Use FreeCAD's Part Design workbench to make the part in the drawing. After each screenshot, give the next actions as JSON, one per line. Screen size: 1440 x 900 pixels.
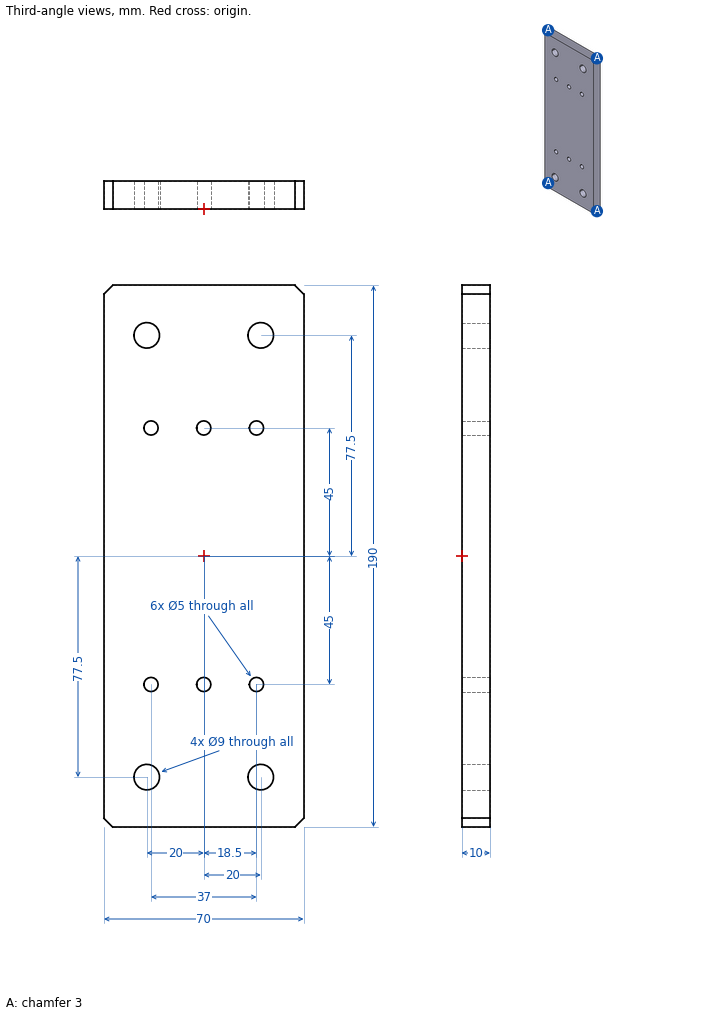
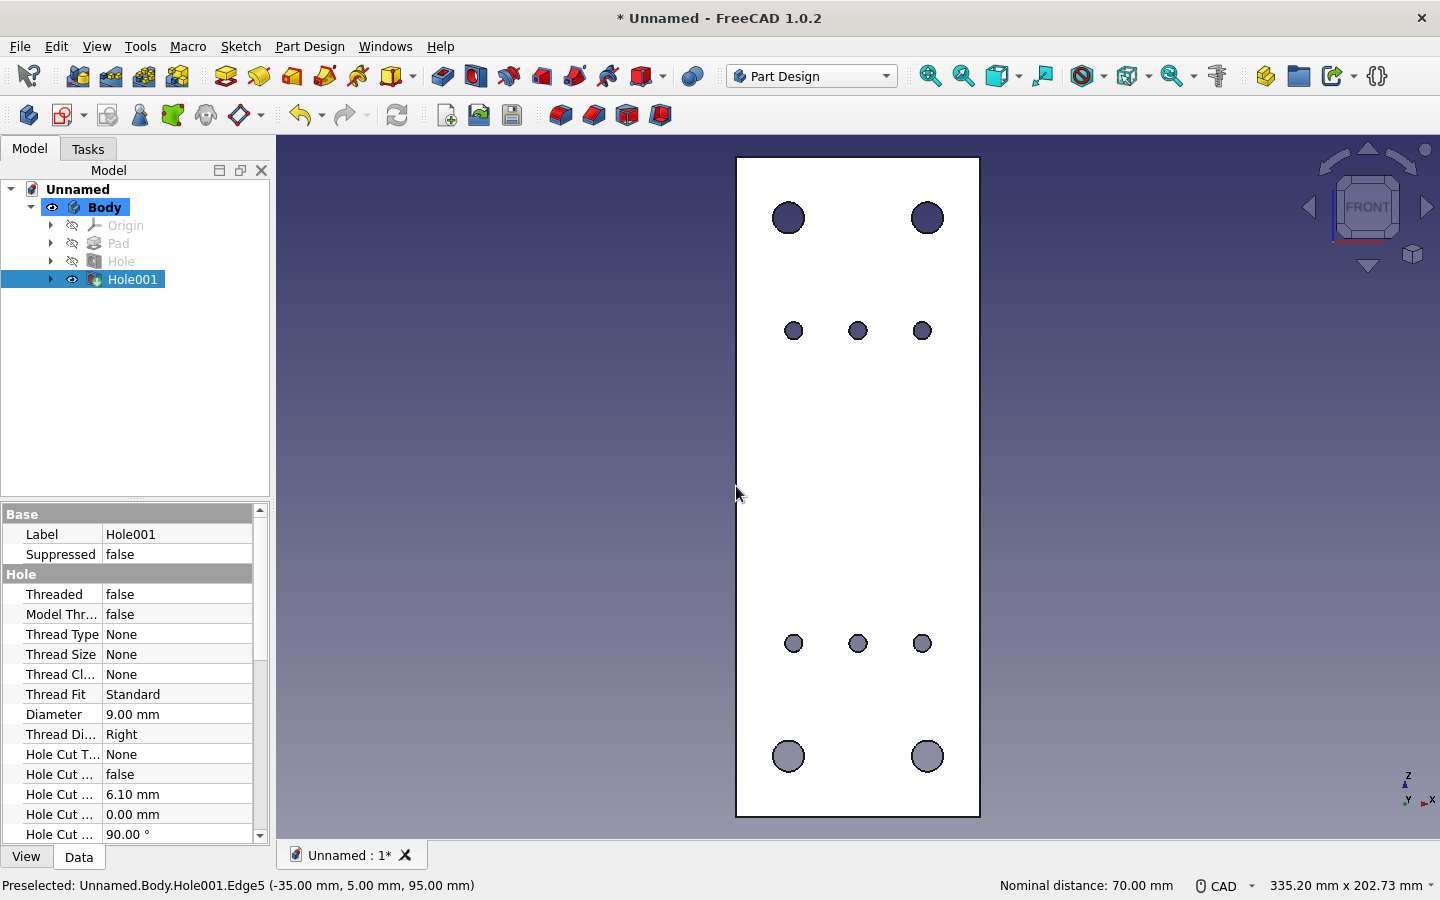
{"action": "key", "text": "3"}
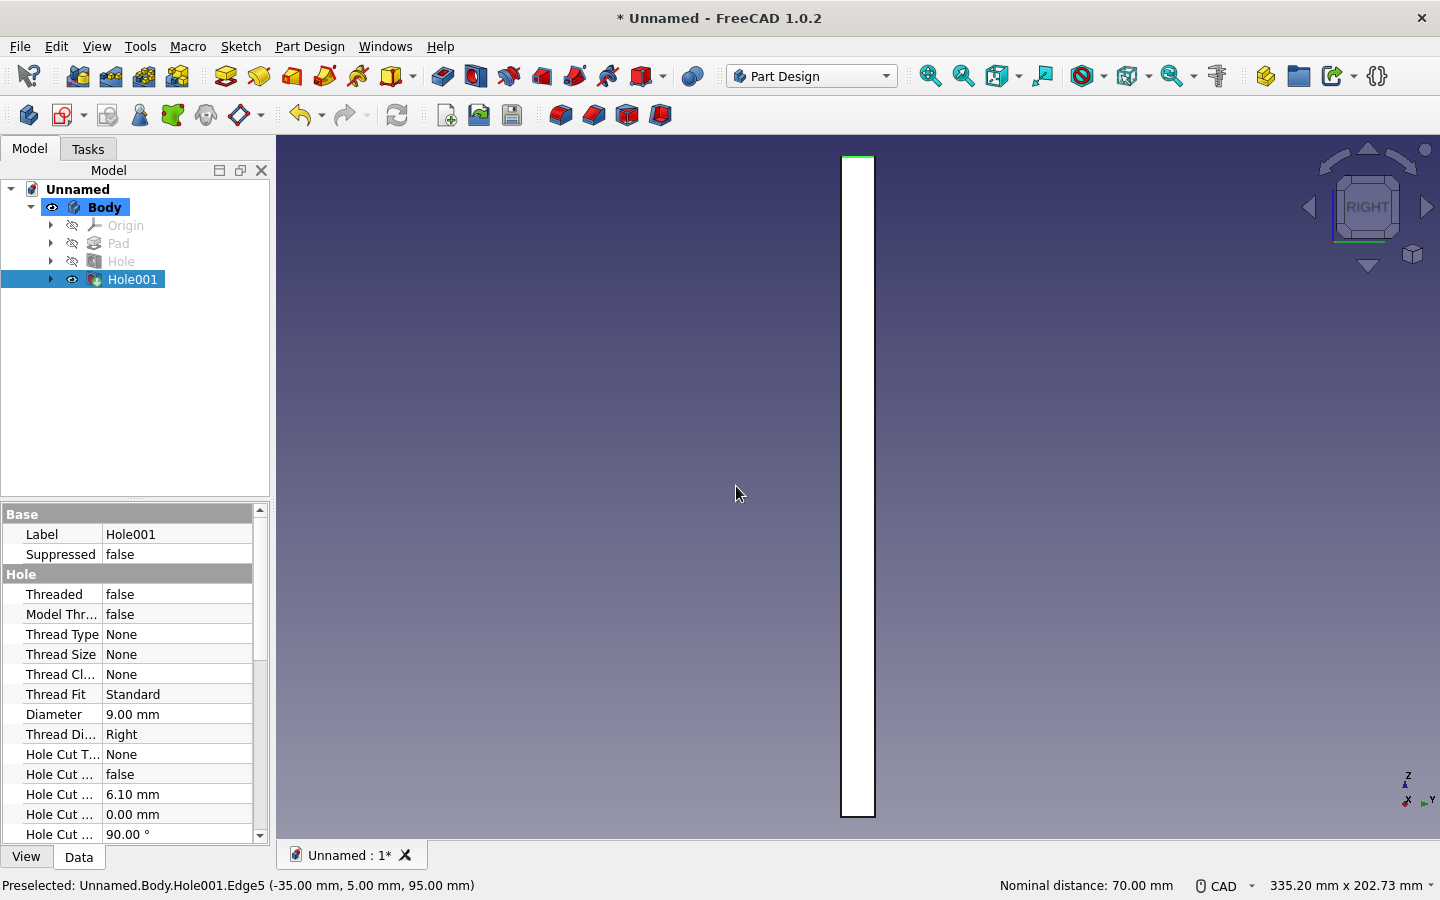
{"action": "key", "text": "5"}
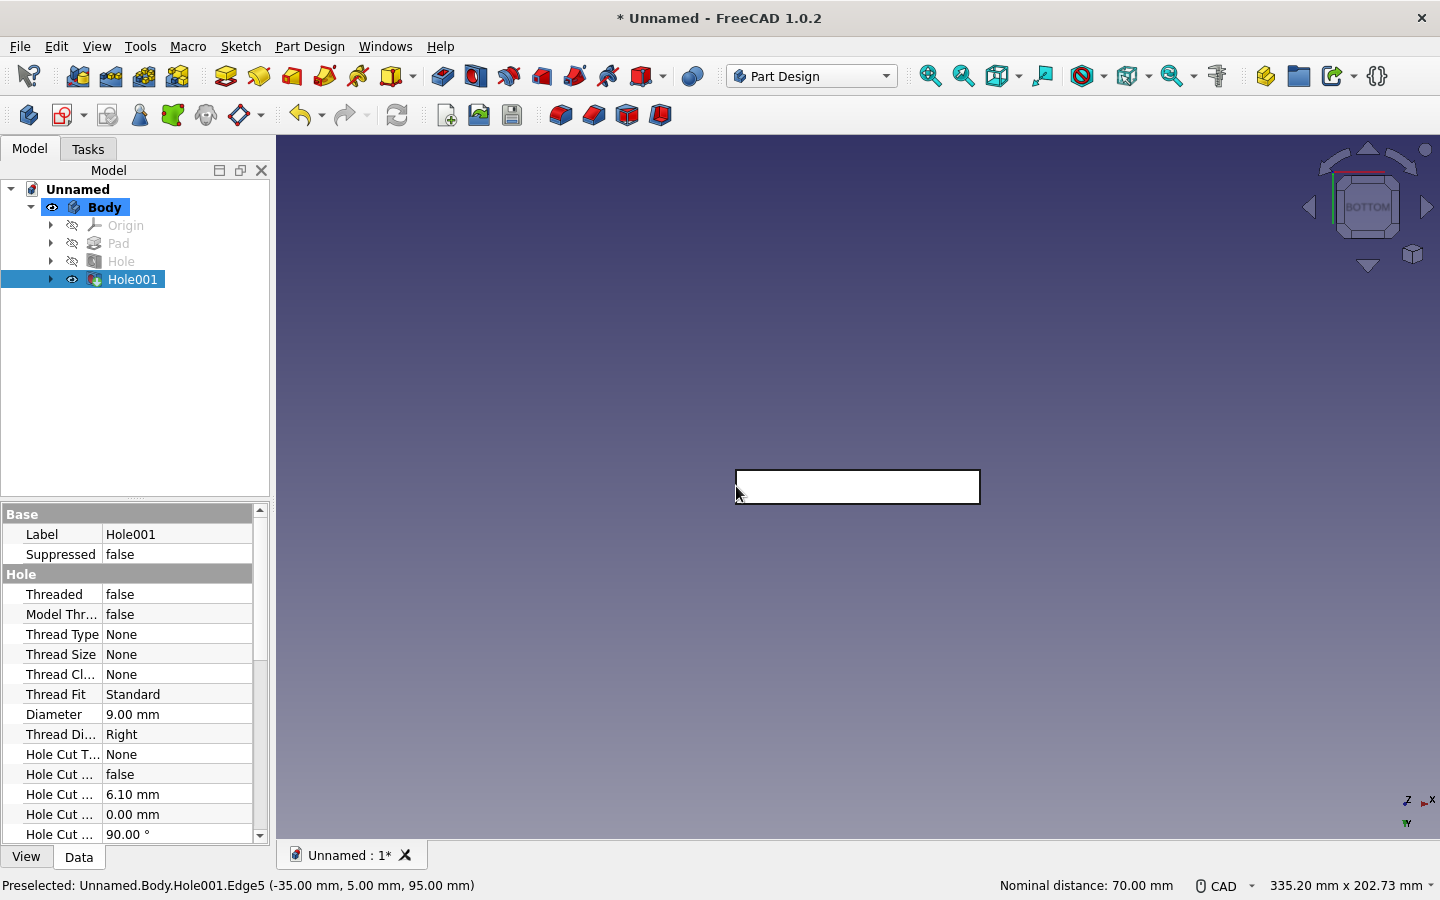
{"action": "left_click", "coordinate": [931, 76]}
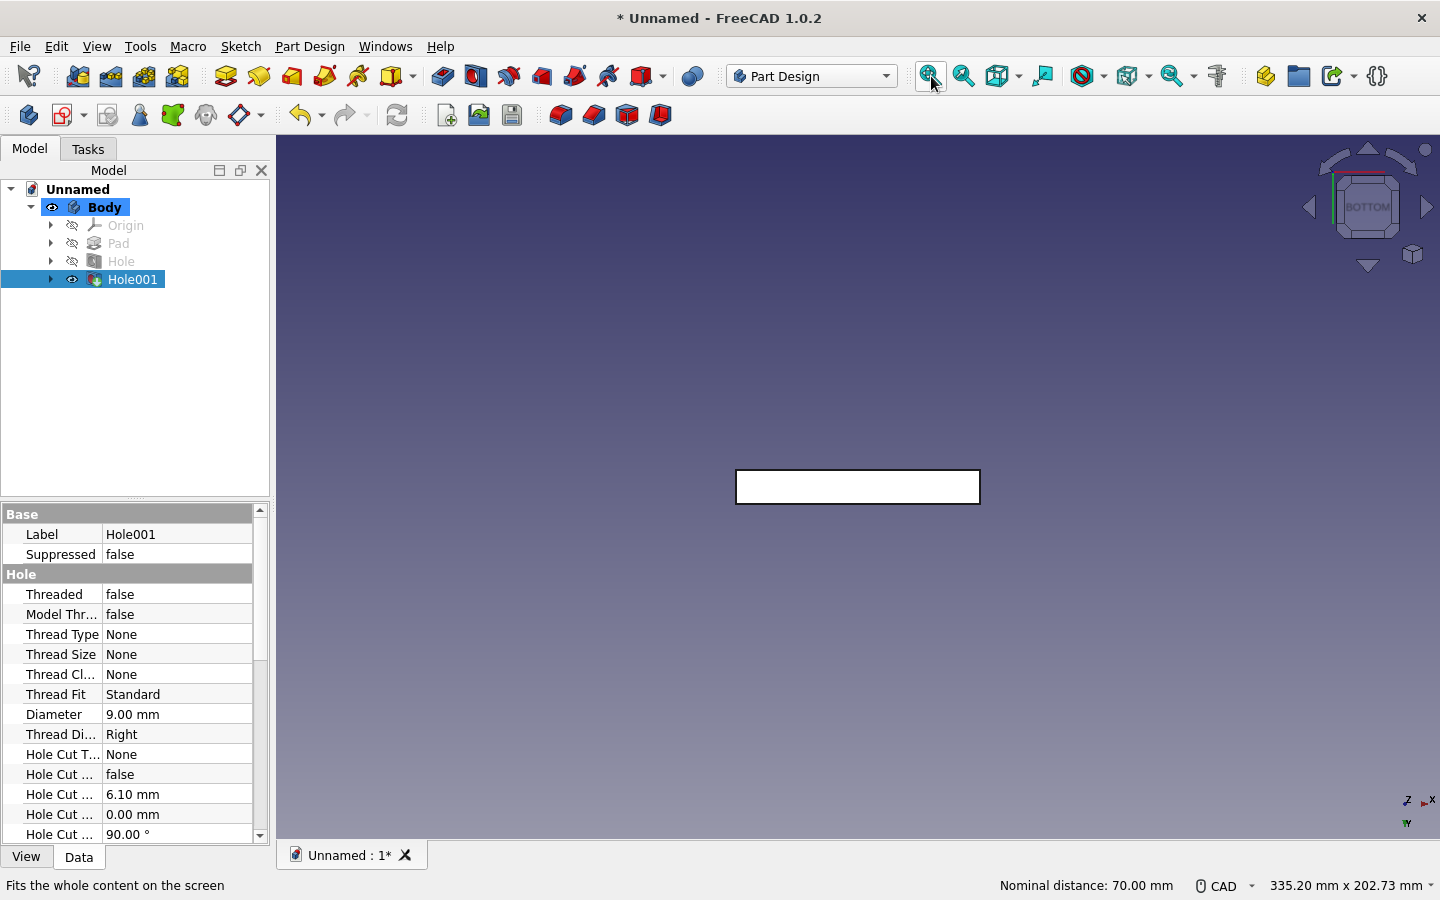
{"action": "left_click", "coordinate": [736, 486], "text": "ctrl"}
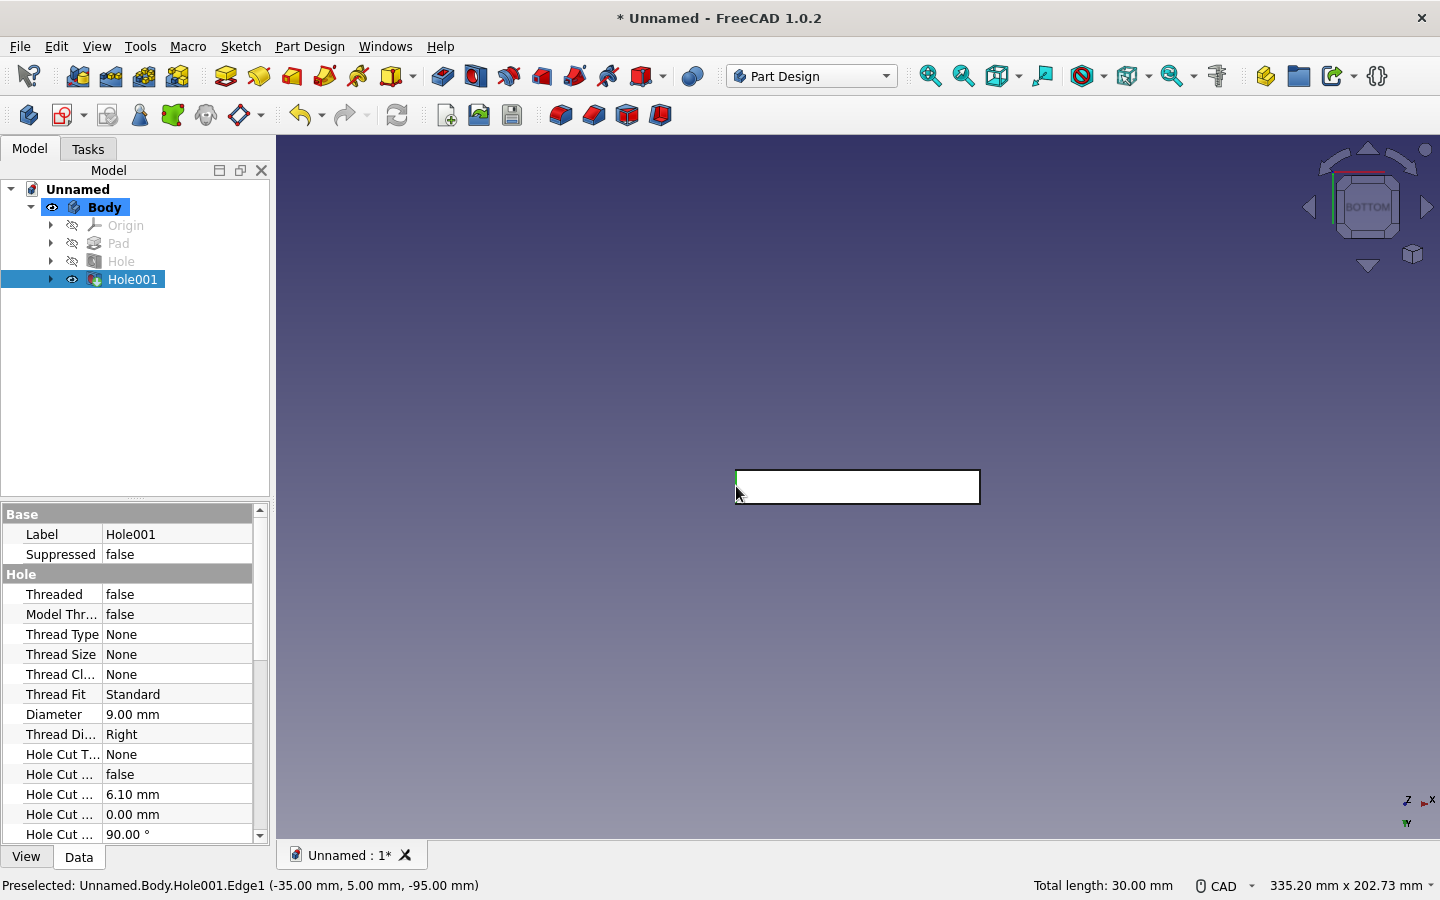
{"action": "left_click", "coordinate": [980, 486], "text": "ctrl"}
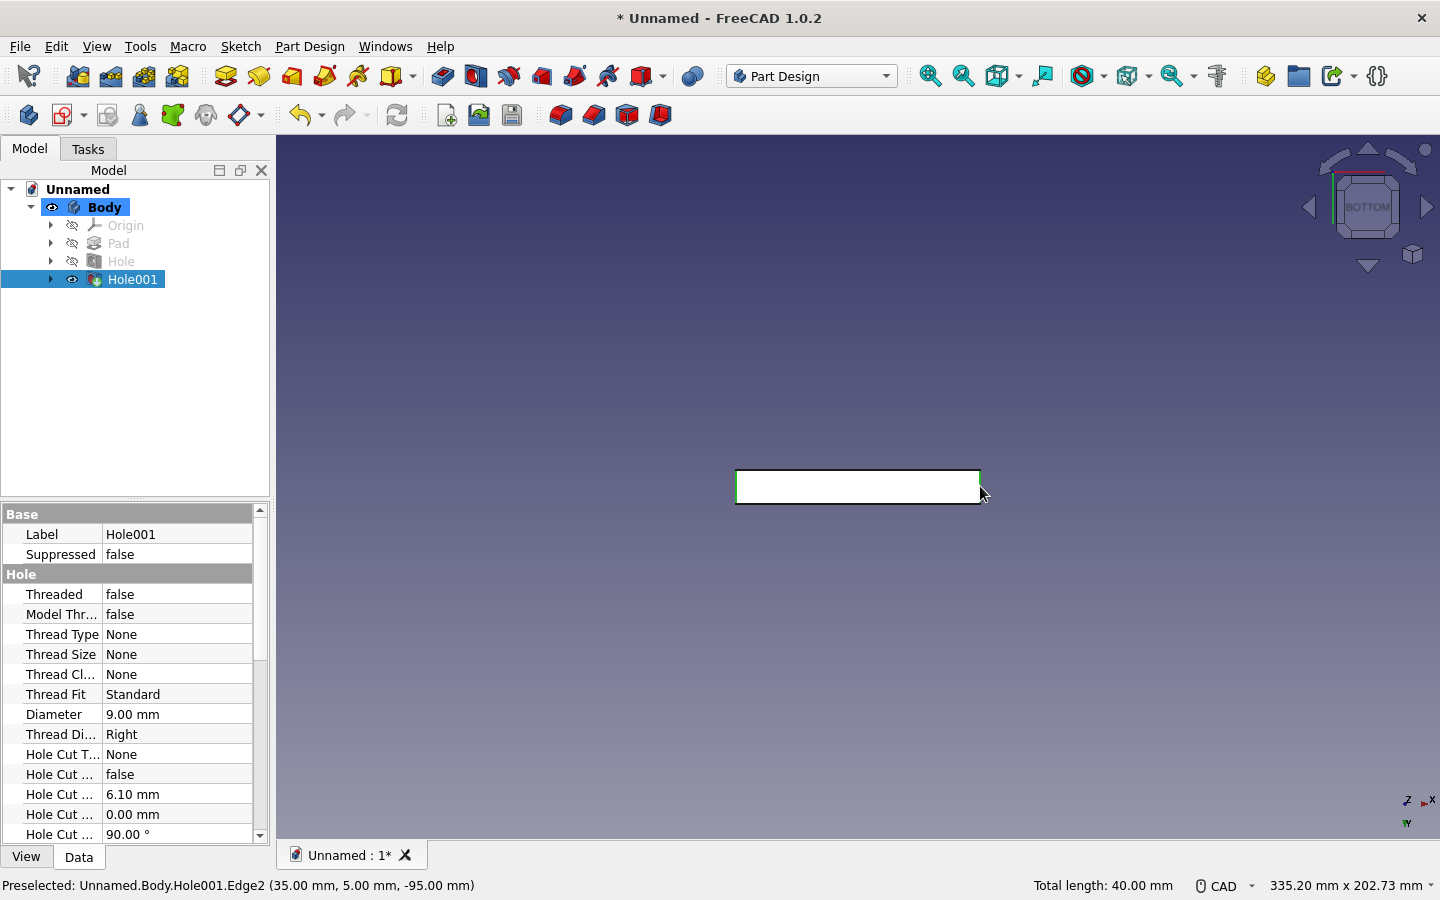
{"action": "left_click", "coordinate": [594, 116]}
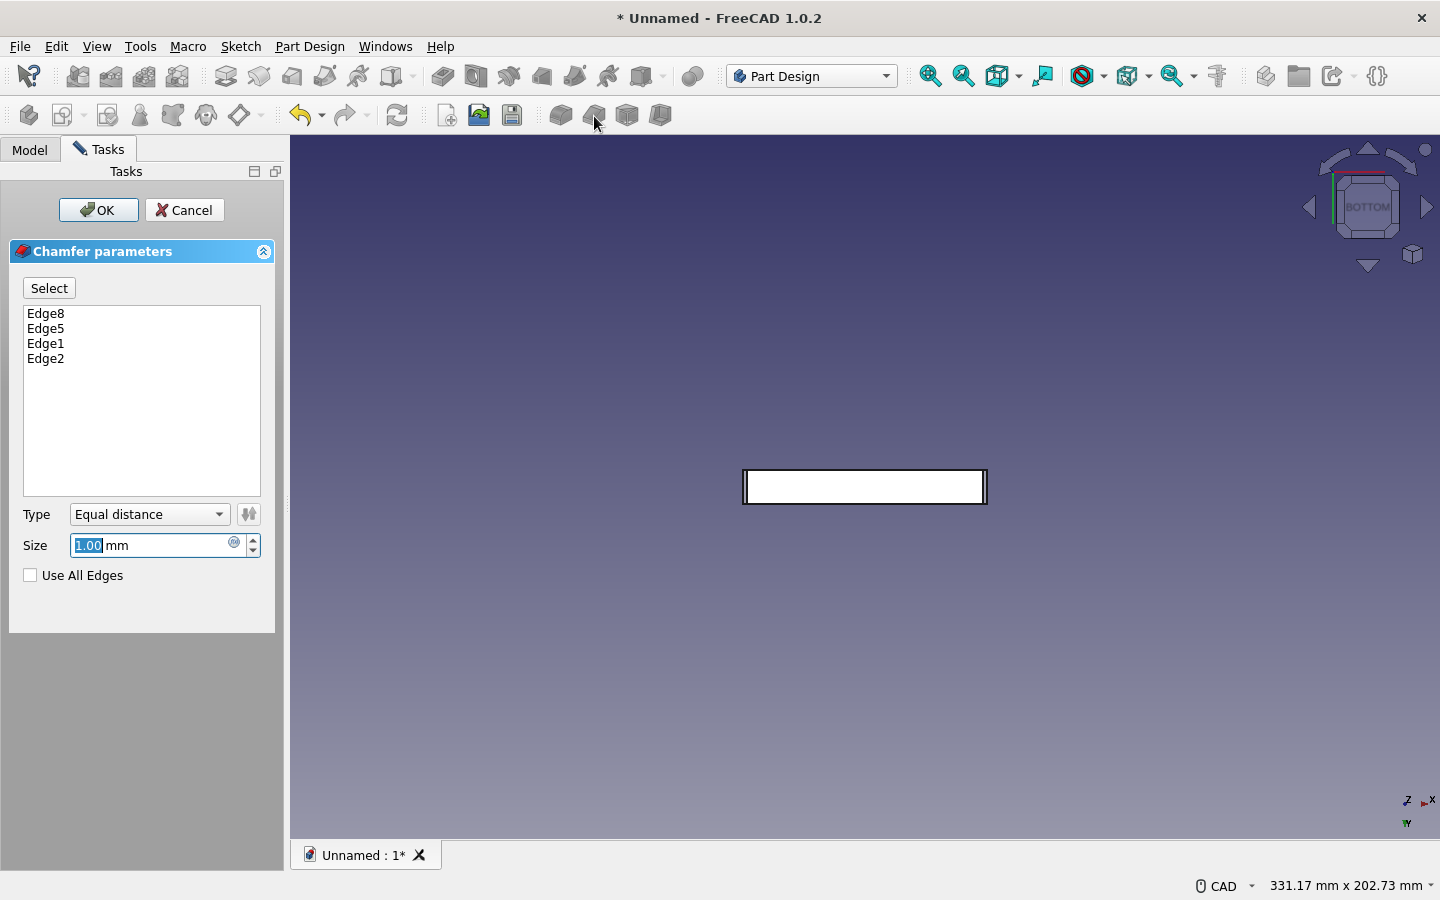
{"action": "type", "text": "3"}
{"action": "key", "text": "Tab"}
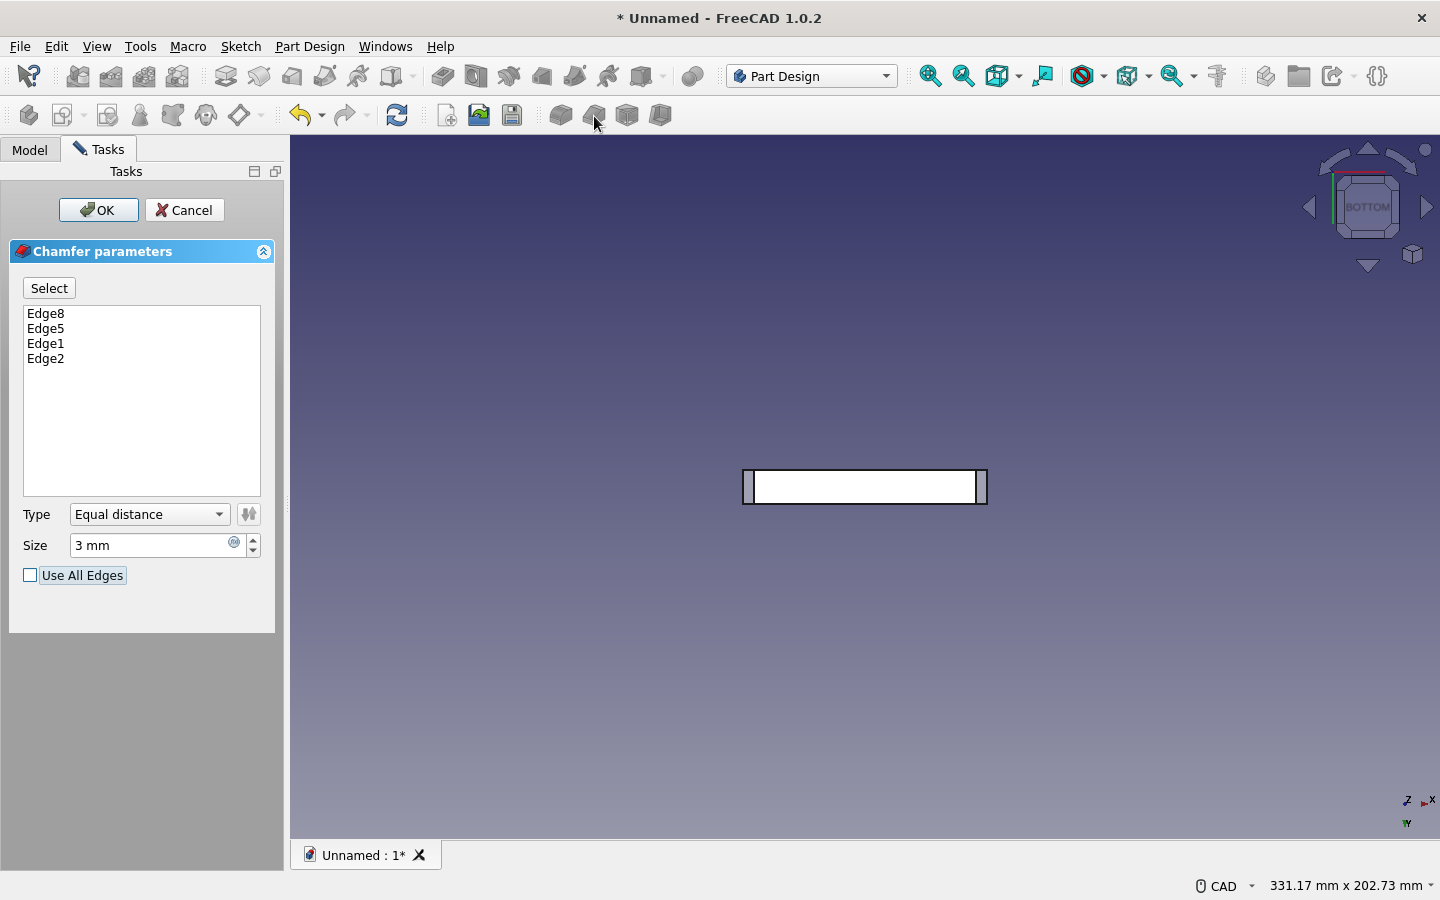
{"action": "left_click", "coordinate": [99, 210]}